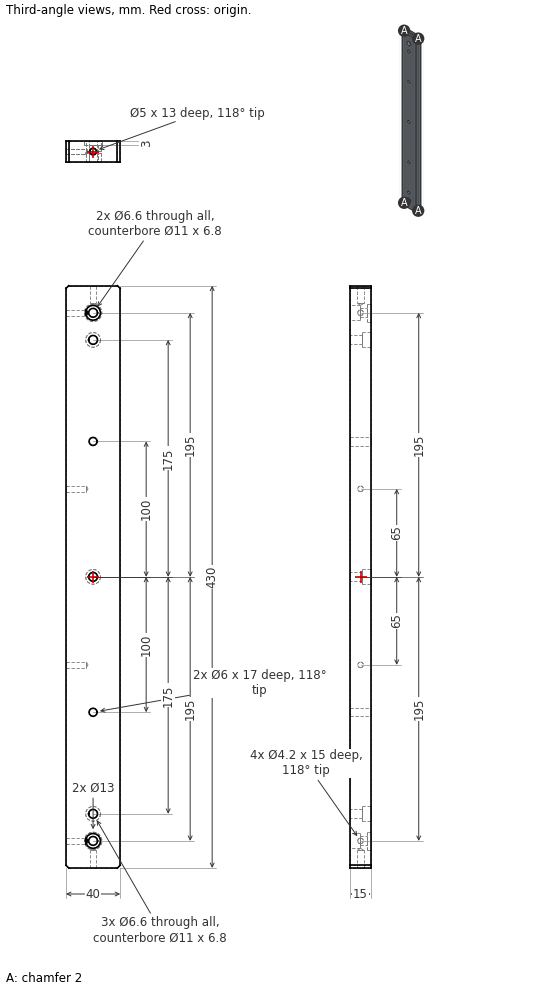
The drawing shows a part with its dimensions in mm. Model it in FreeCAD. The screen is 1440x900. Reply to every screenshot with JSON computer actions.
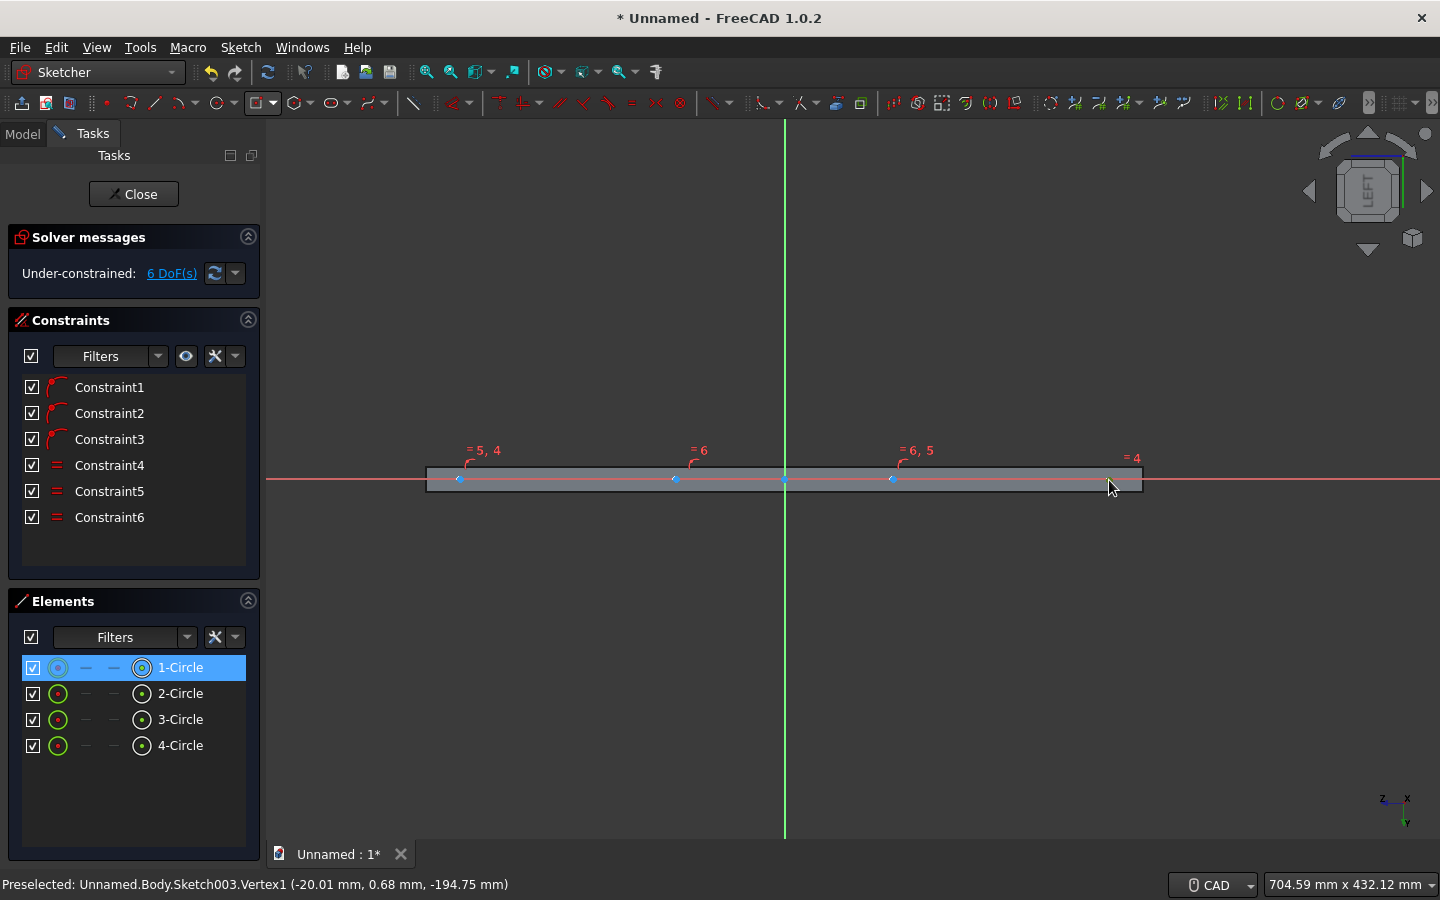
{"action": "left_click", "coordinate": [364, 479]}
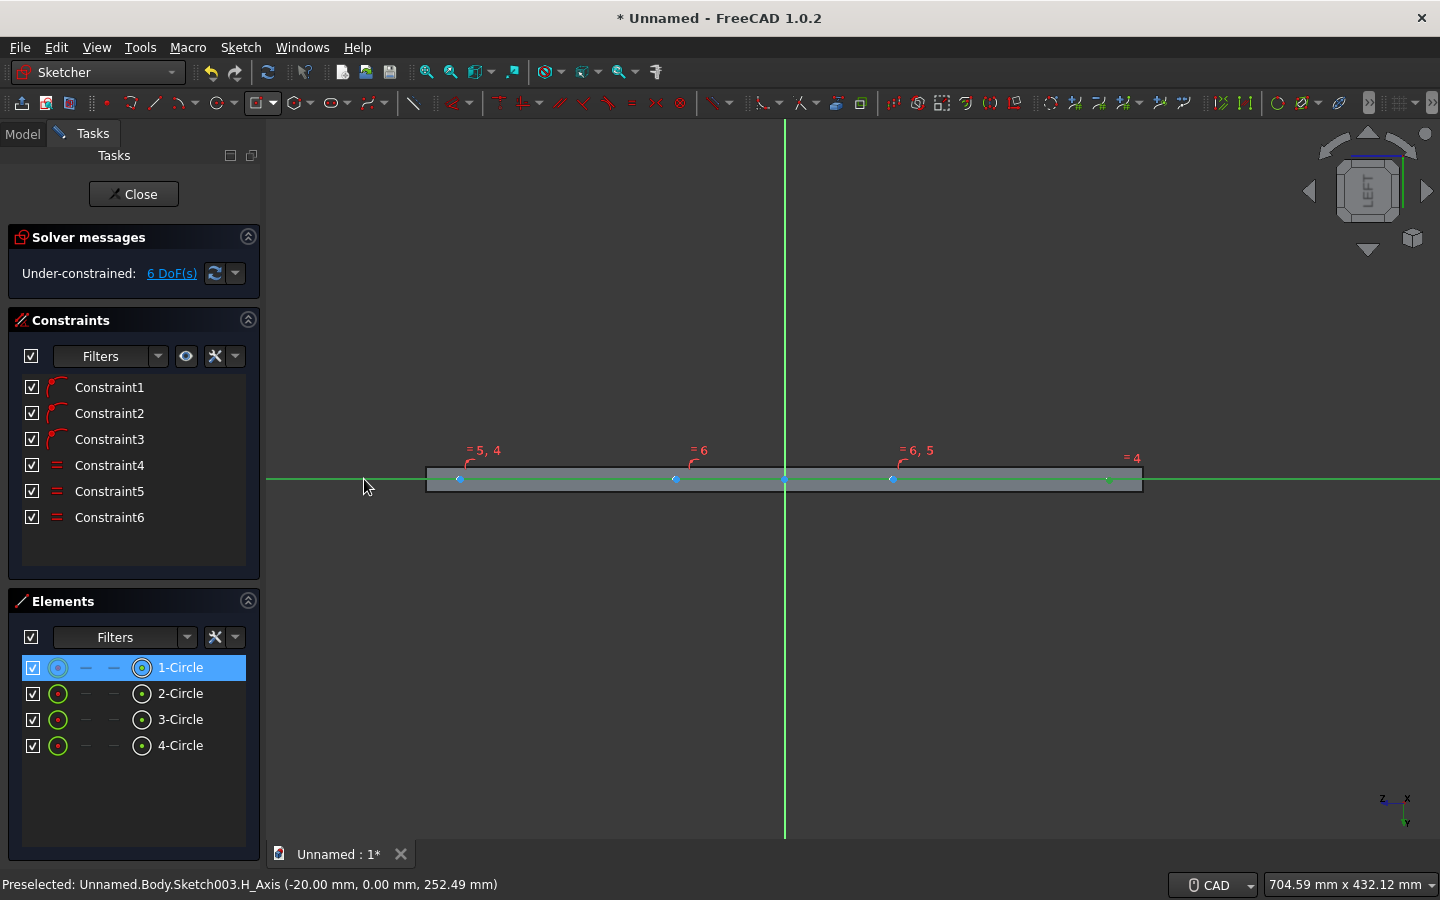
{"action": "left_click", "coordinate": [500, 104]}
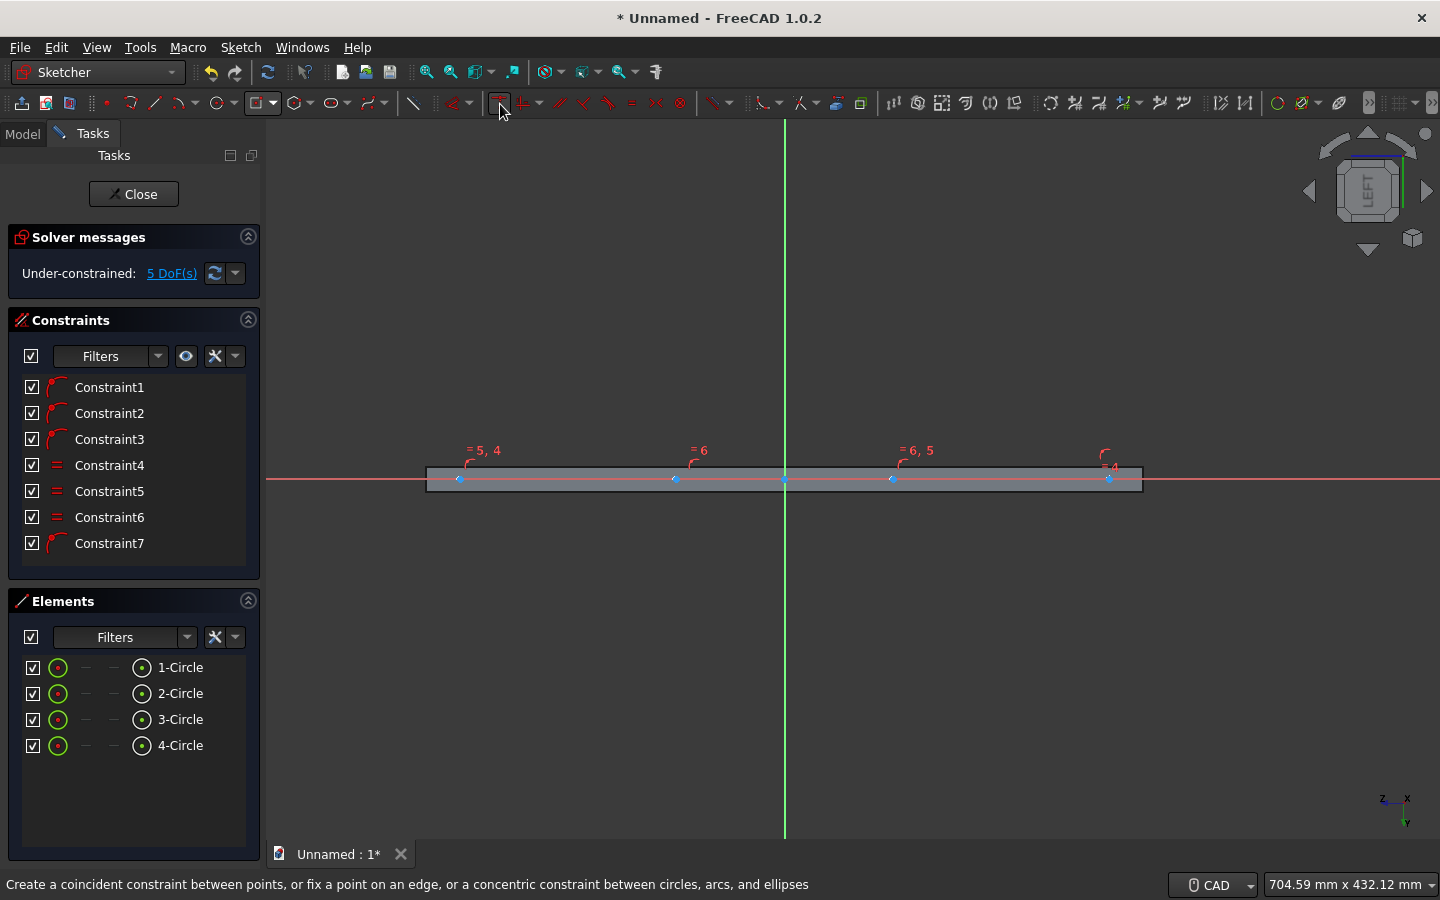
{"action": "key", "text": "d"}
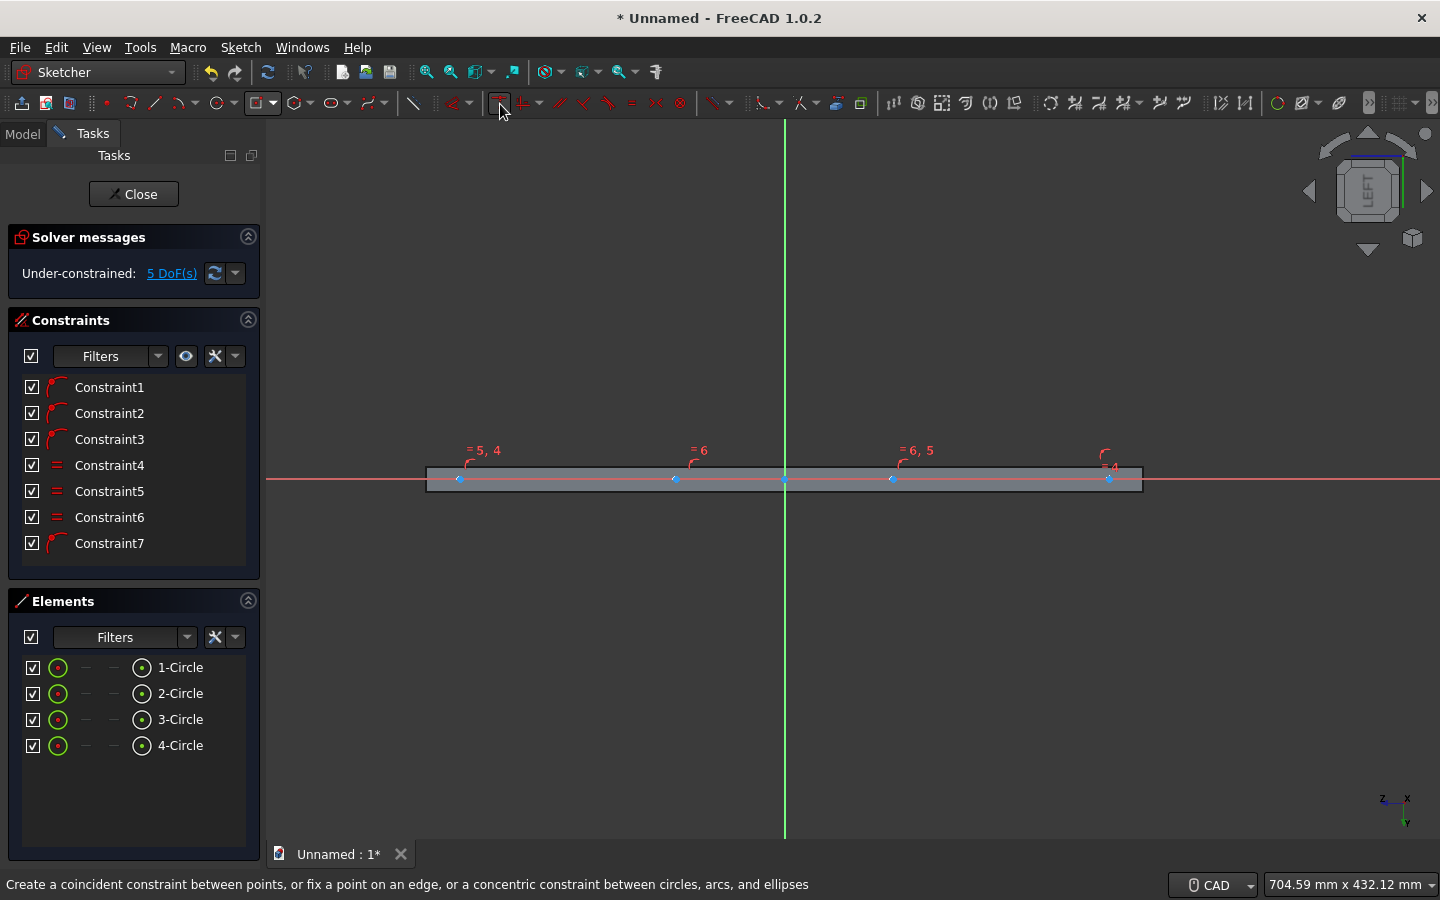
{"action": "scroll", "coordinate": [1111, 481], "scroll_direction": "up", "scroll_amount": 9}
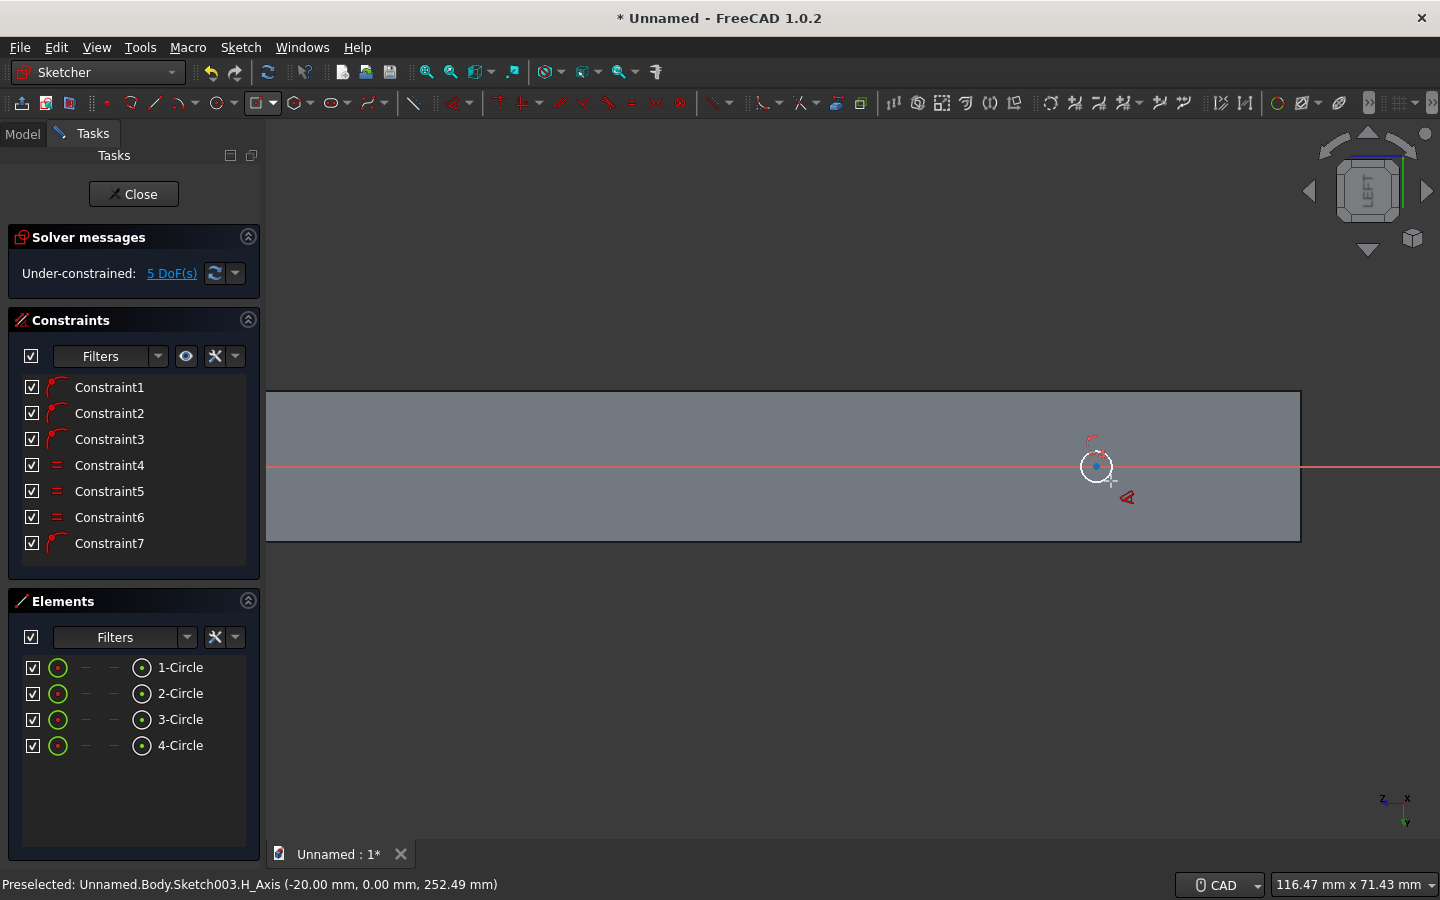
{"action": "left_click", "coordinate": [1107, 478]}
{"action": "left_click", "coordinate": [1129, 501]}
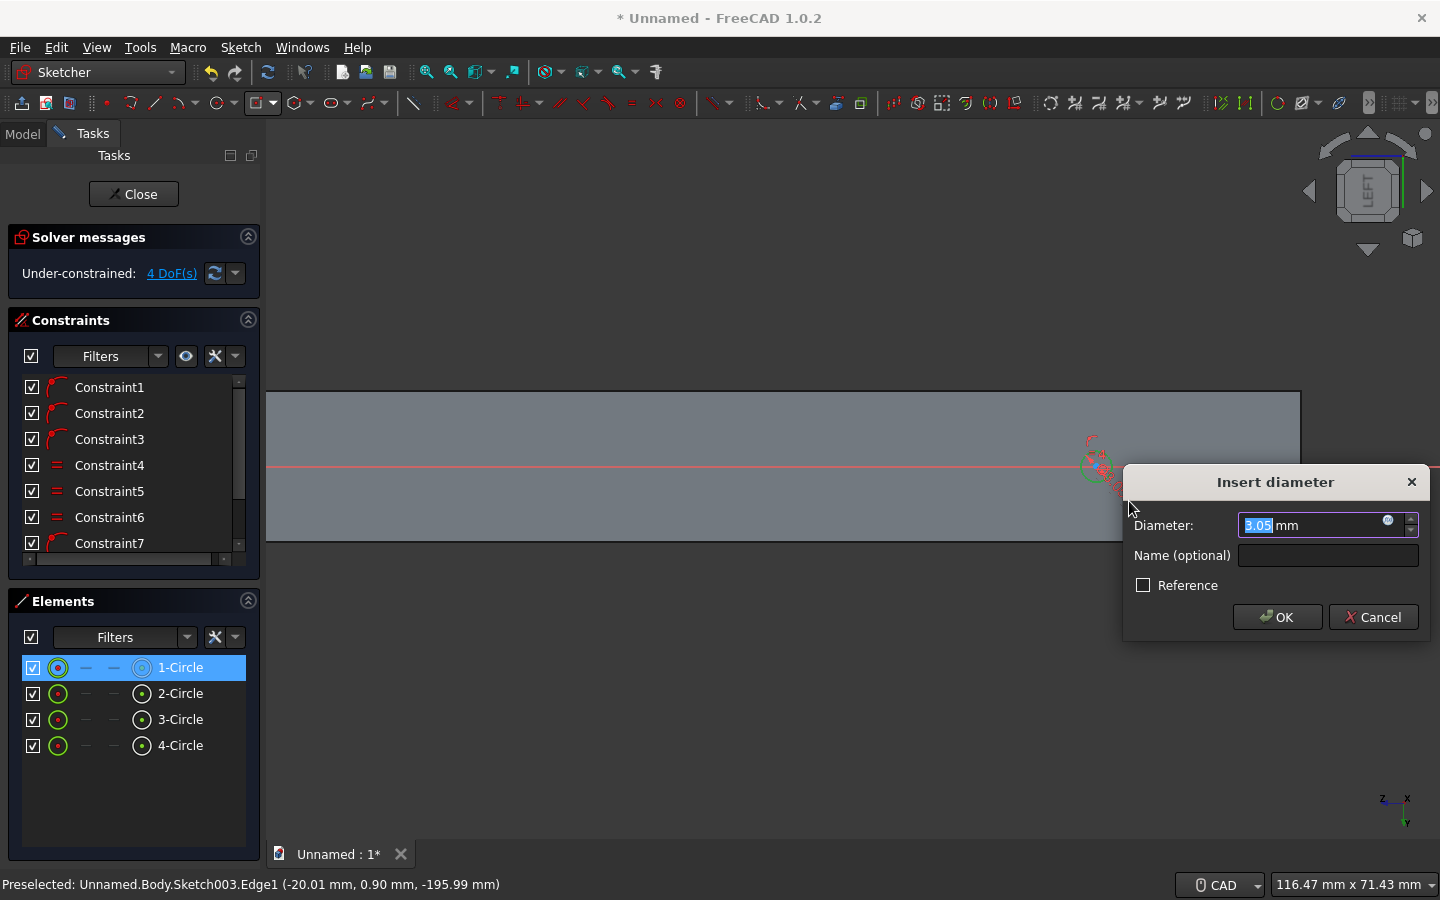
{"action": "type", "text": "4.2"}
{"action": "key", "text": "Return"}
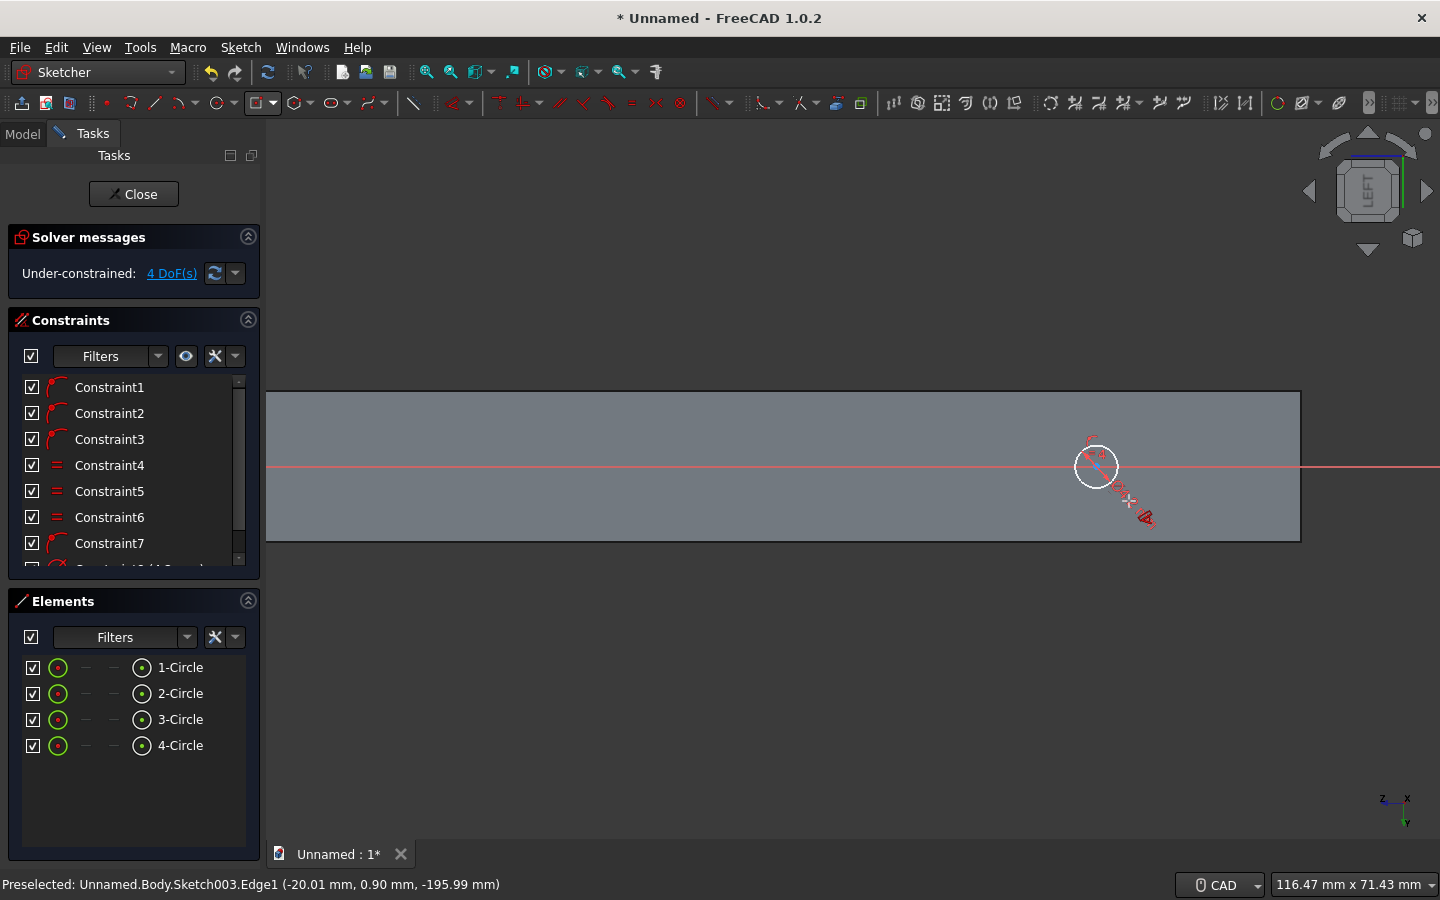
{"action": "scroll", "coordinate": [1111, 481], "scroll_direction": "down", "scroll_amount": 9}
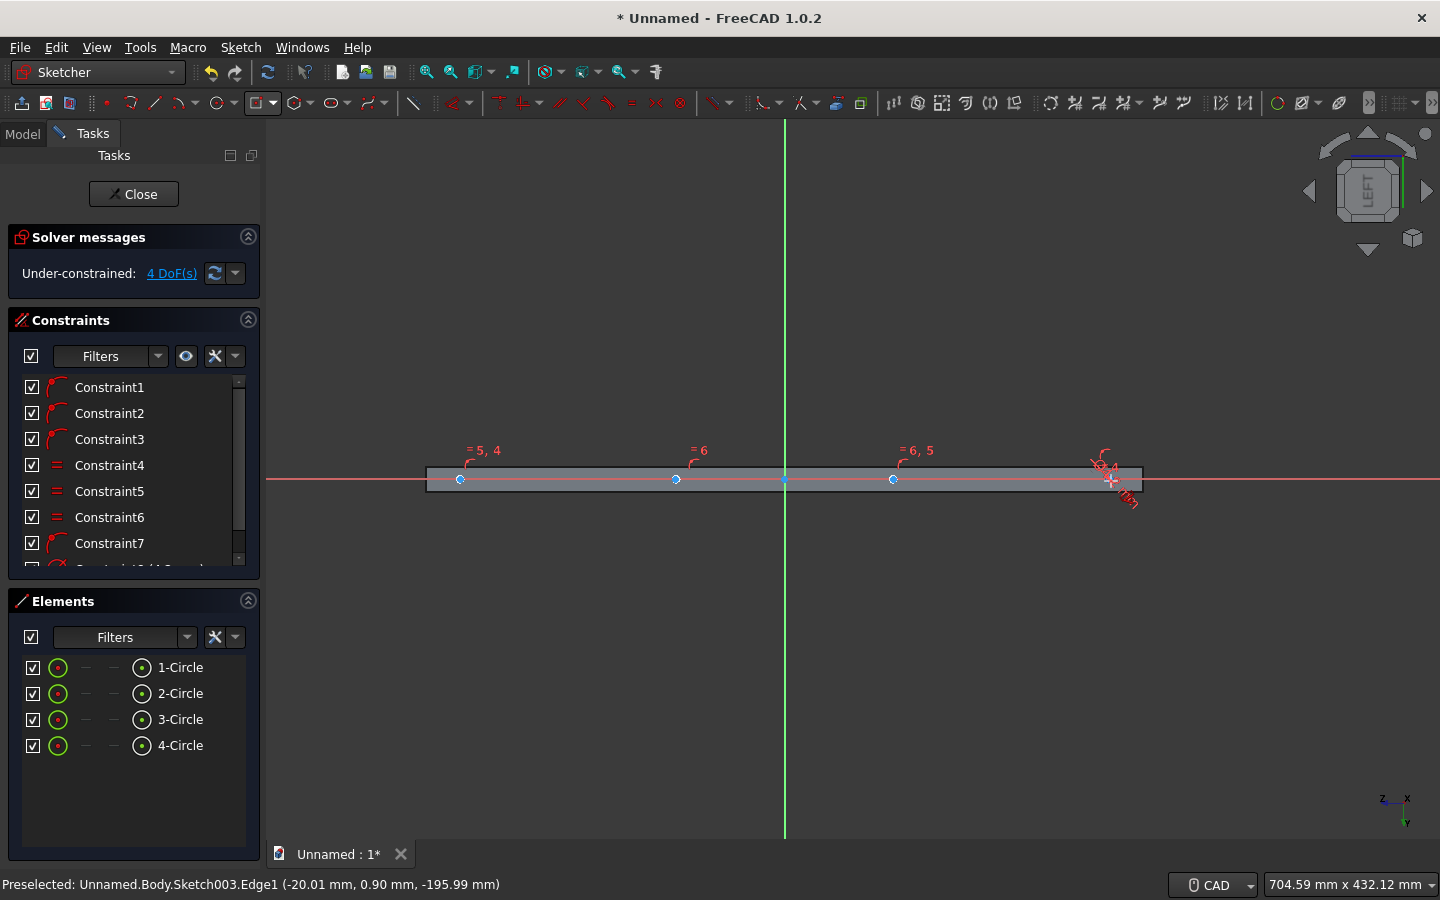
{"action": "left_click", "coordinate": [893, 479]}
{"action": "left_click", "coordinate": [839, 513]}